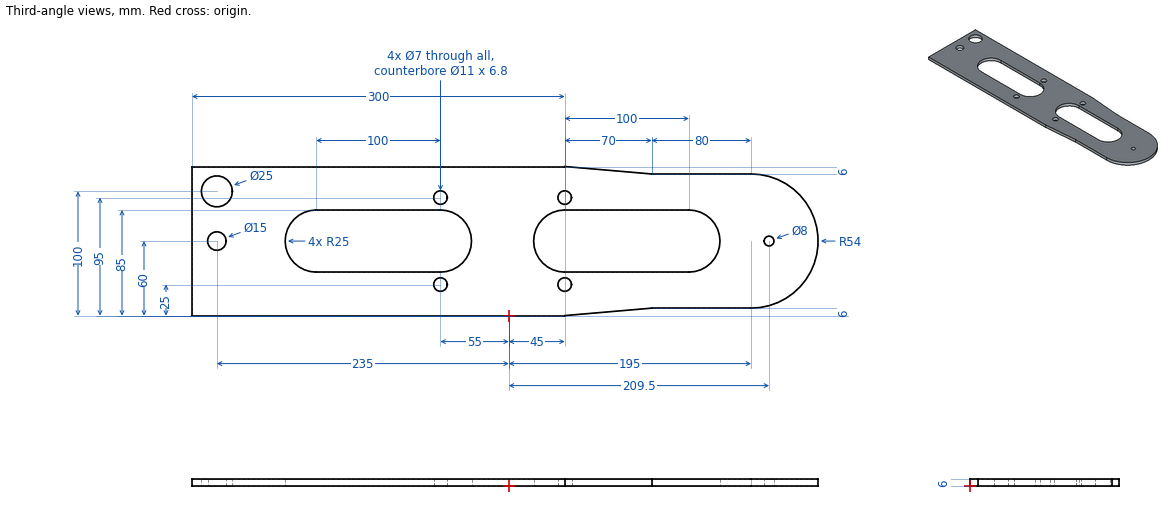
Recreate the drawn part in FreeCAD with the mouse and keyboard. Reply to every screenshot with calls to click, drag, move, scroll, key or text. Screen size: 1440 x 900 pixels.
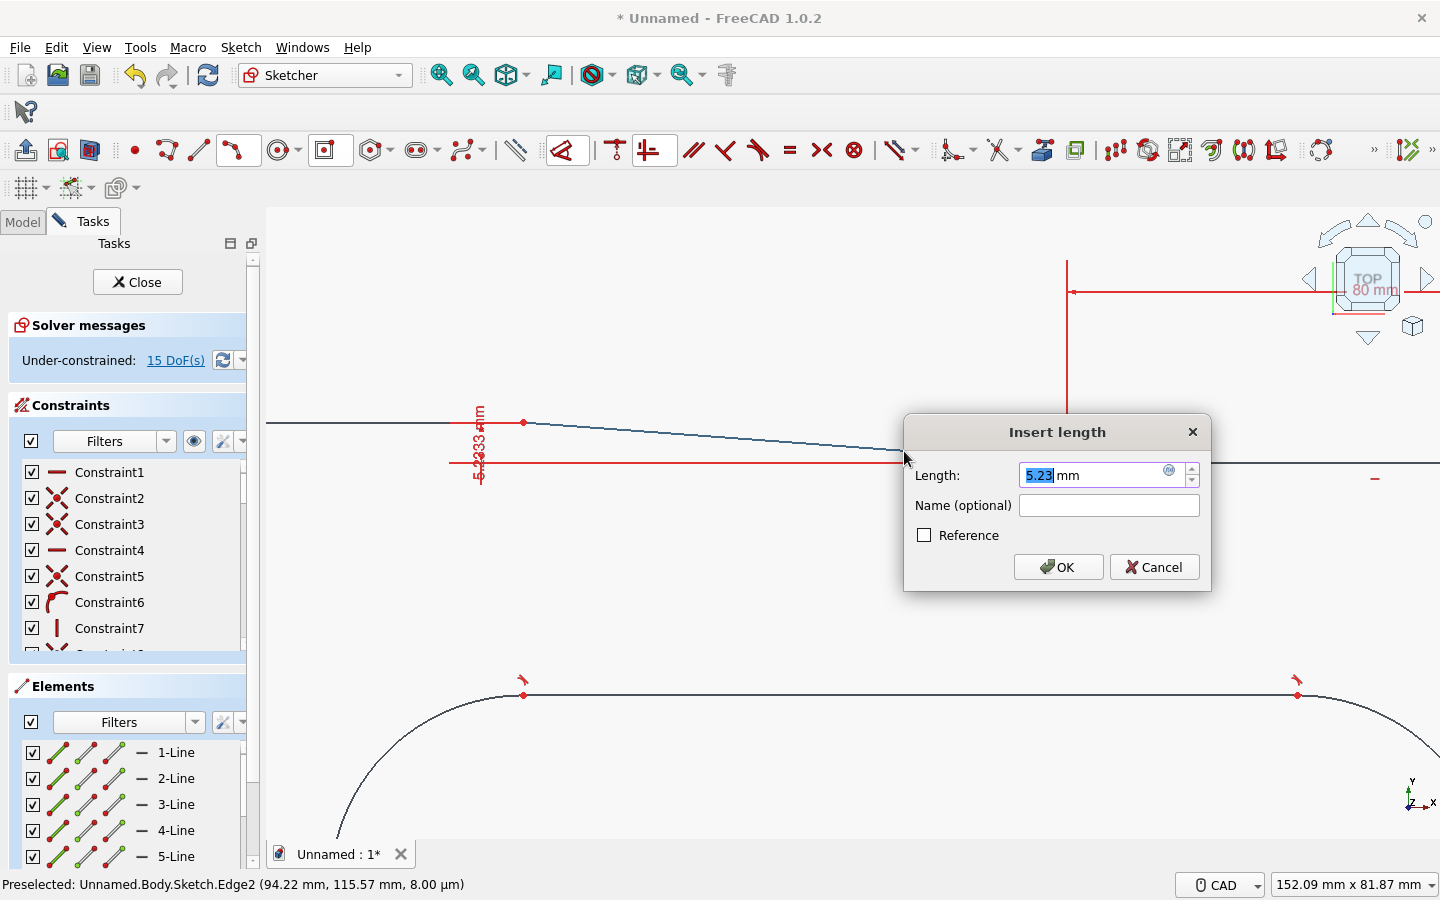
text(6)
key(Return)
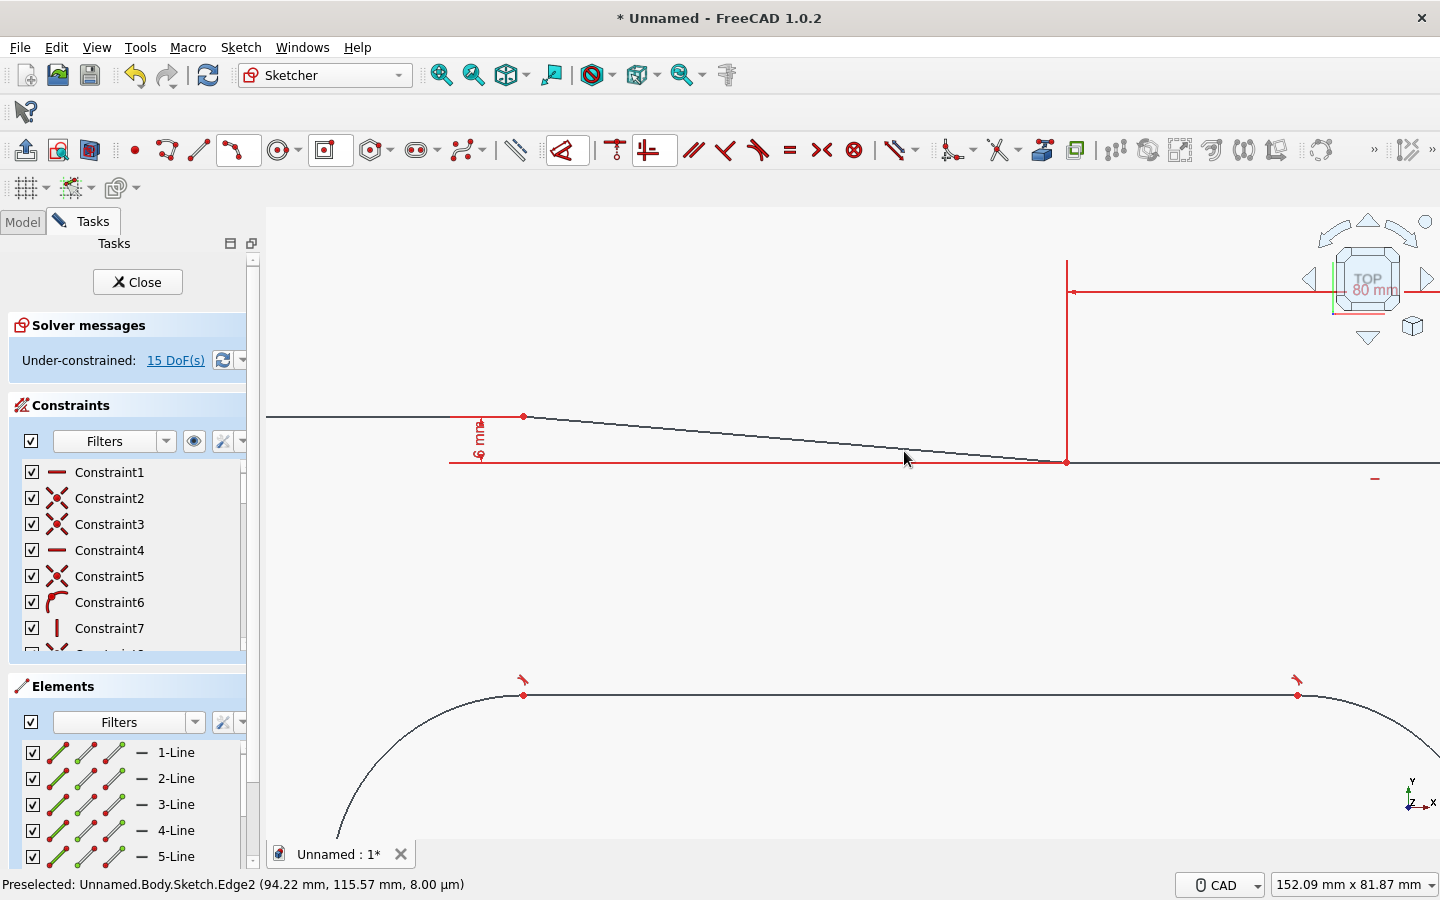
scroll(909, 452, down, 9)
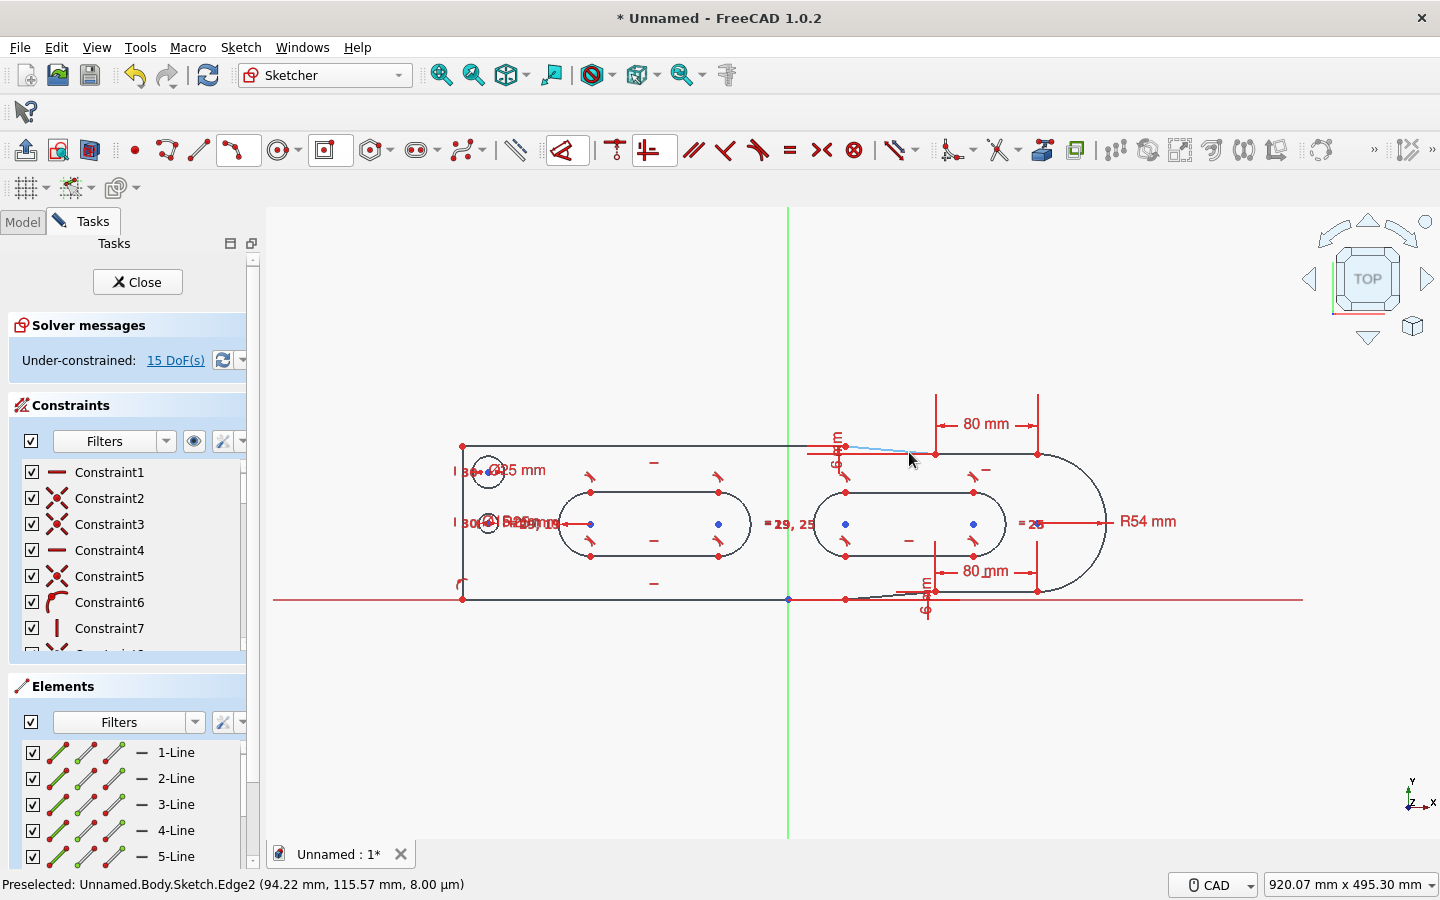
click(488, 523)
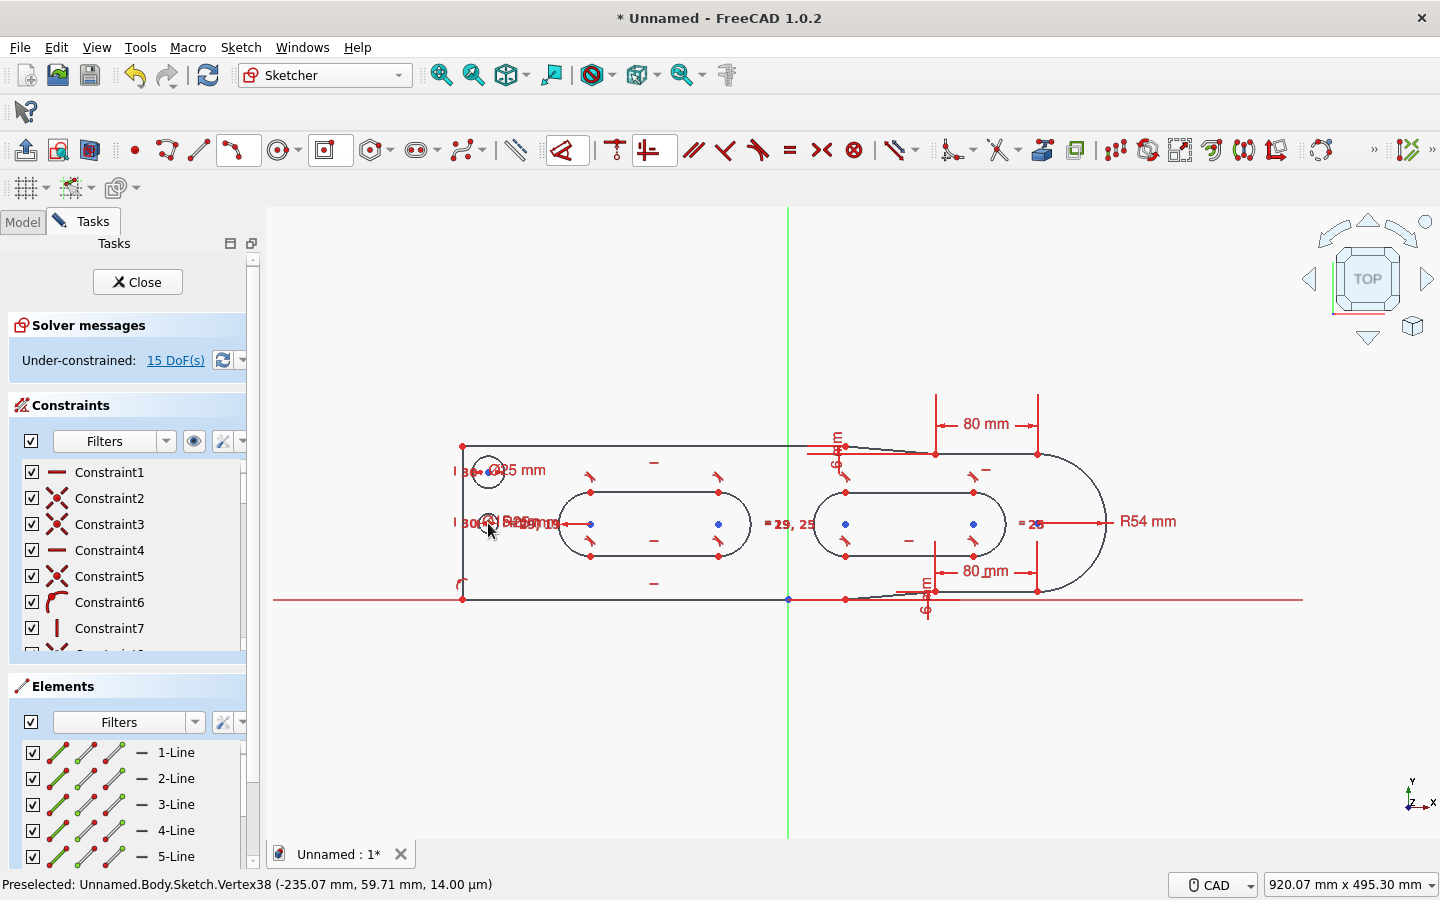
key(i)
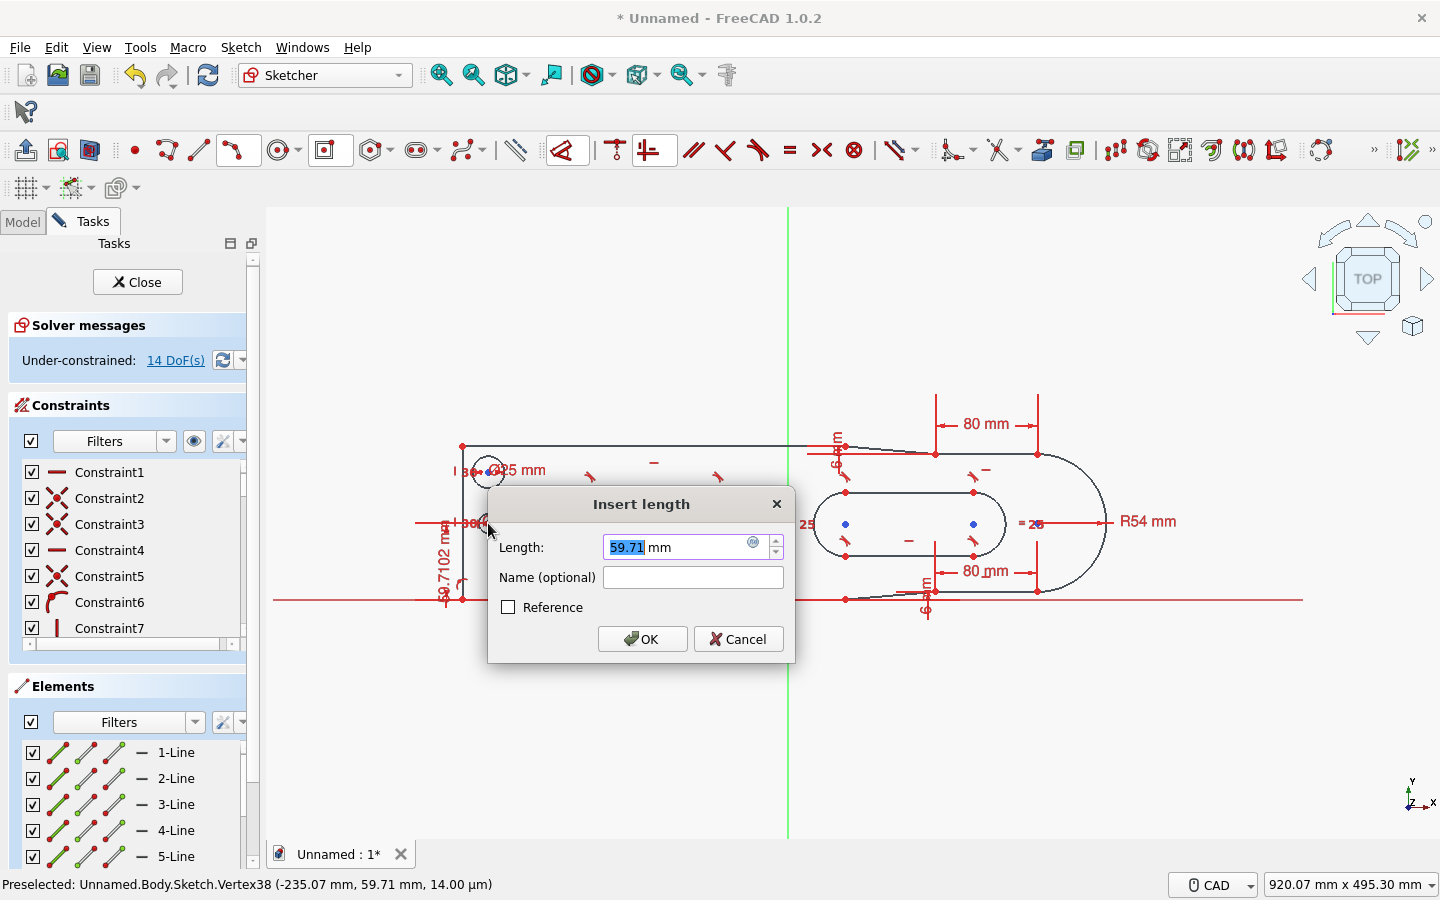
text(60)
key(Return)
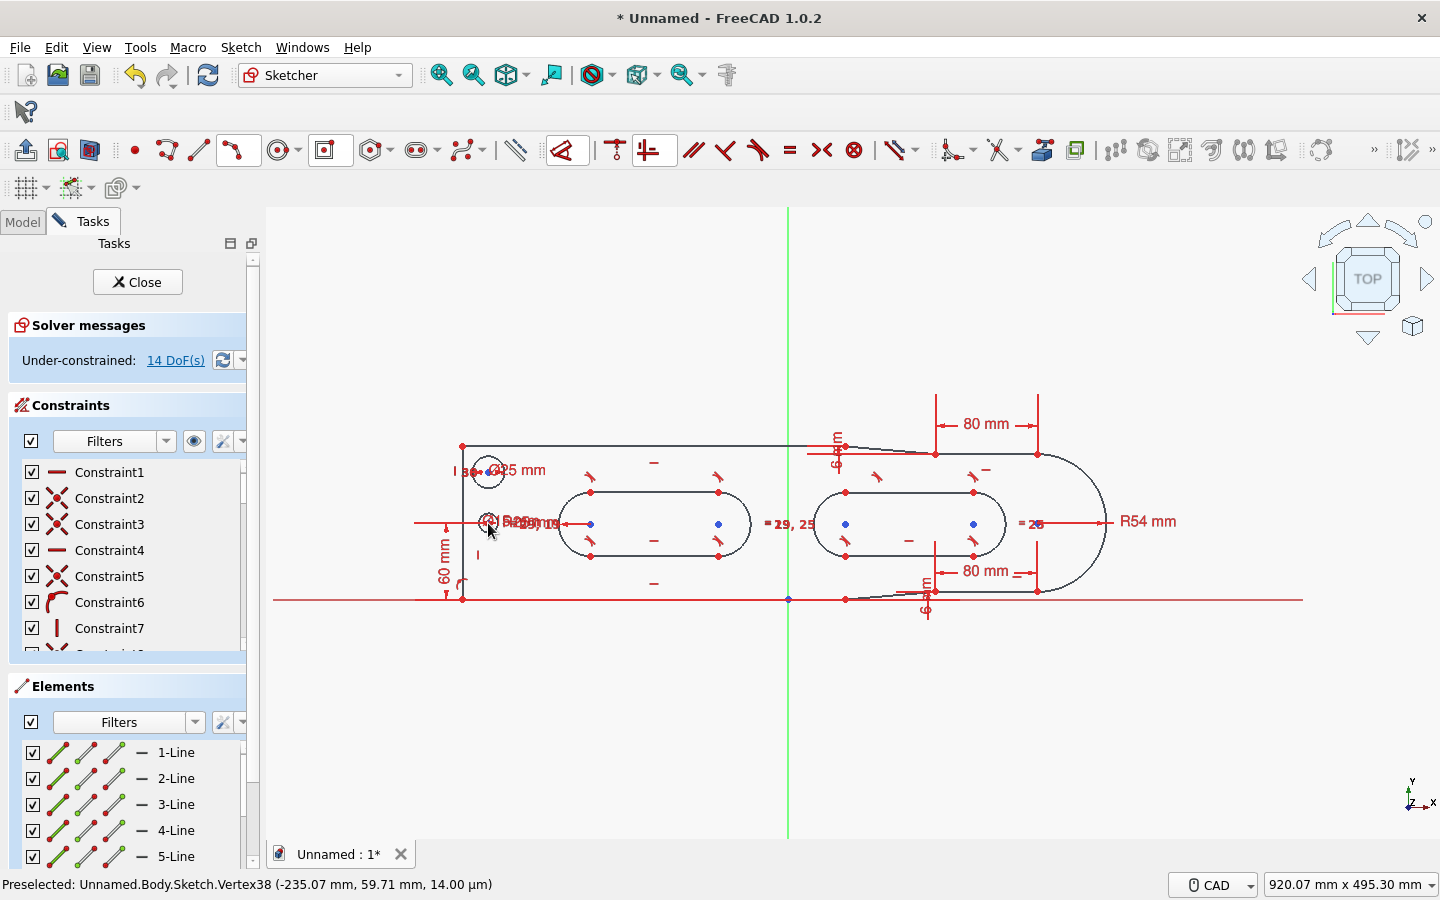
click(731, 446)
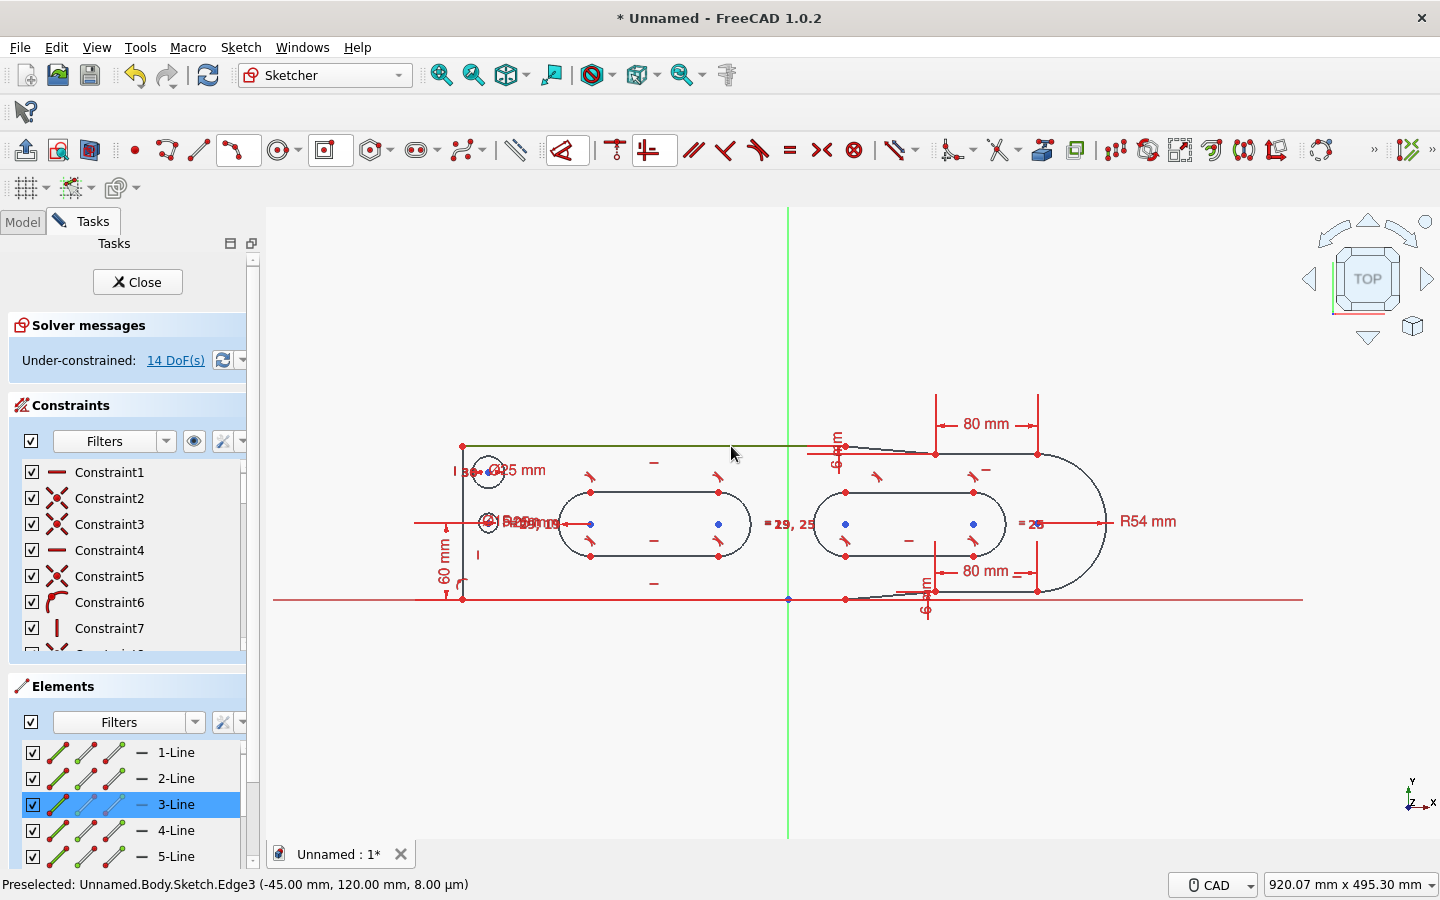
key(l)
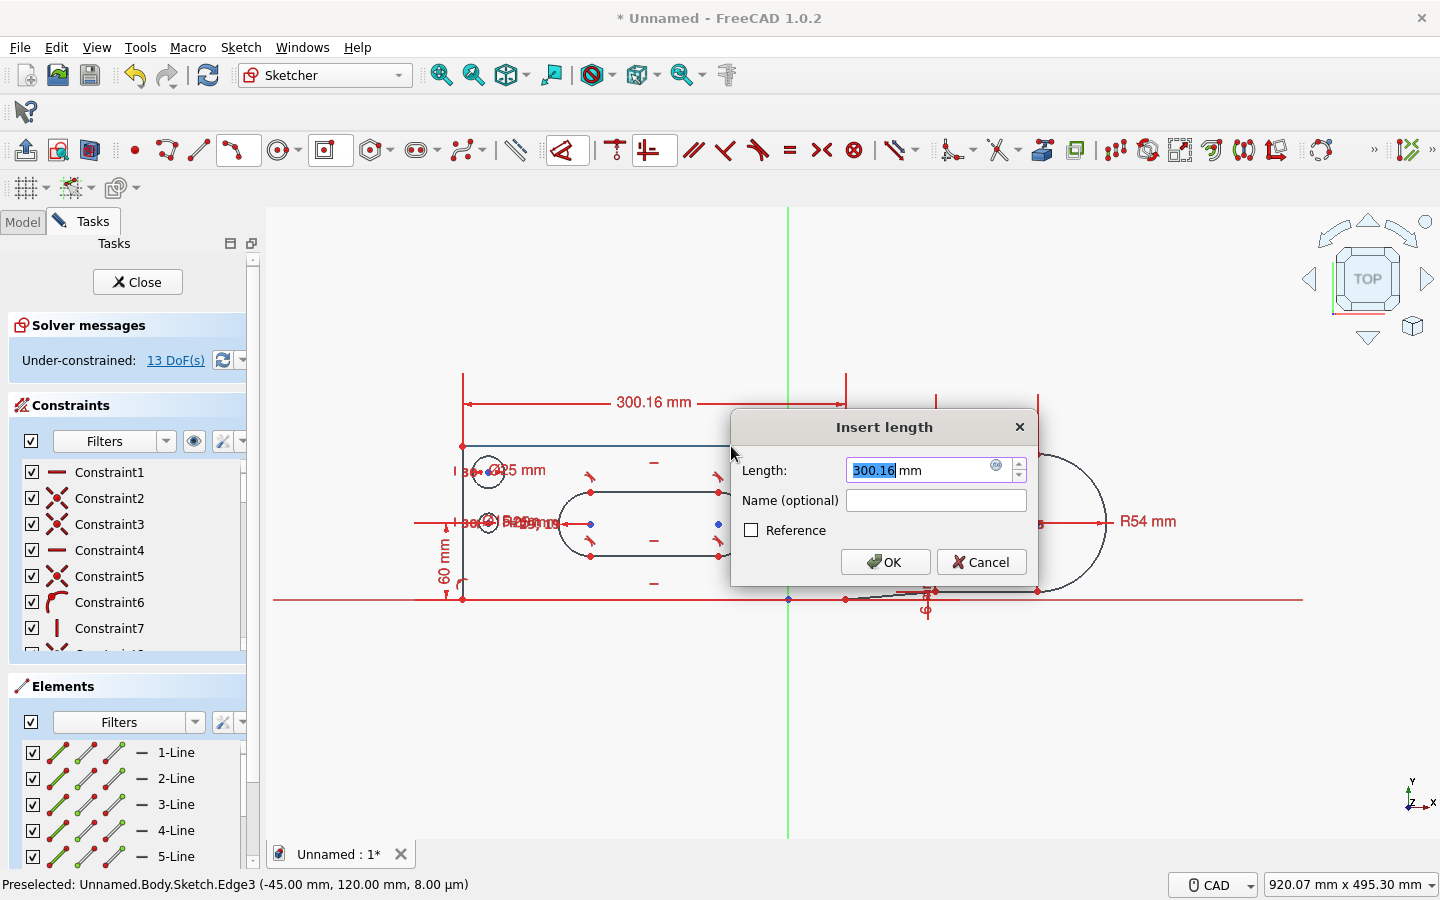
text(300)
key(Return)